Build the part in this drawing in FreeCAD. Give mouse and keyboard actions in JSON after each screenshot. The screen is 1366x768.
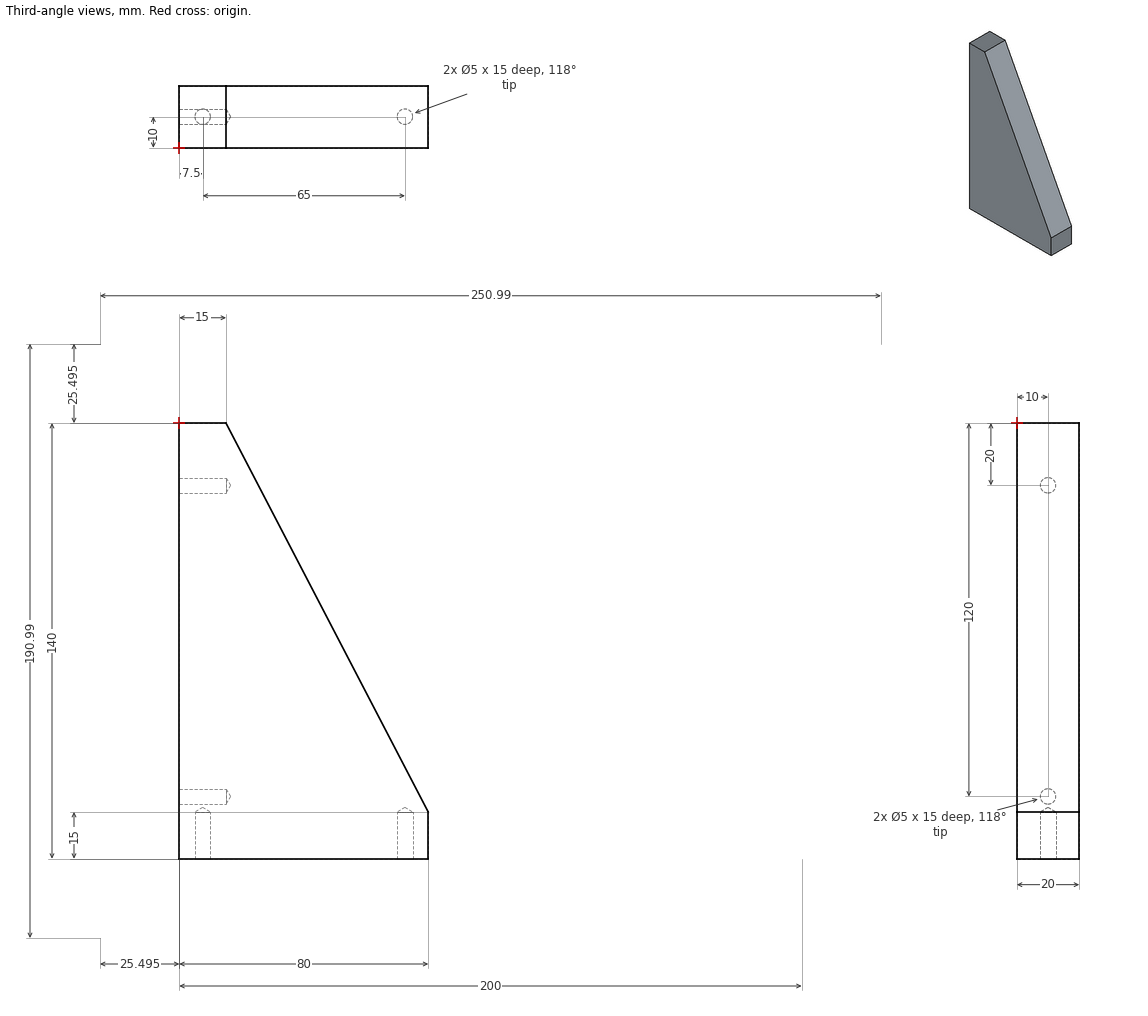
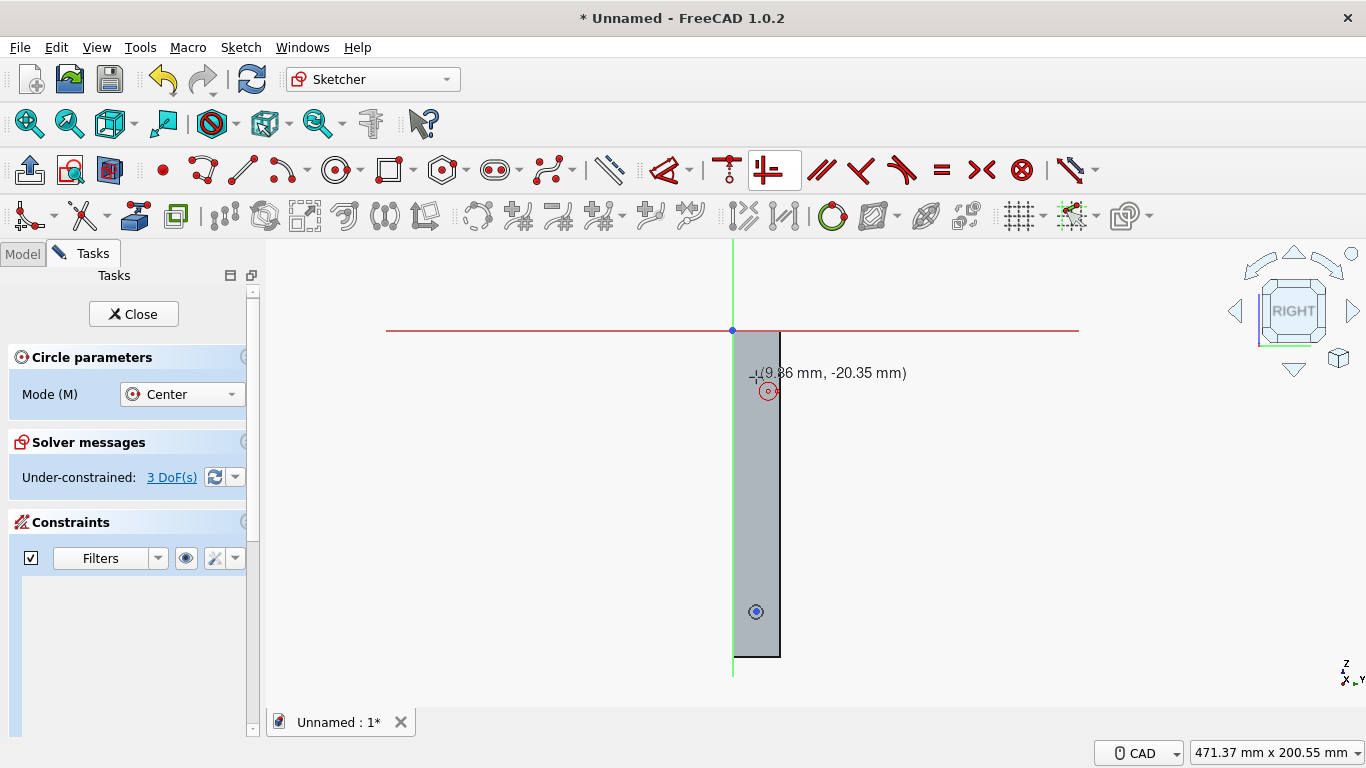
{"action": "left_click", "coordinate": [756, 377]}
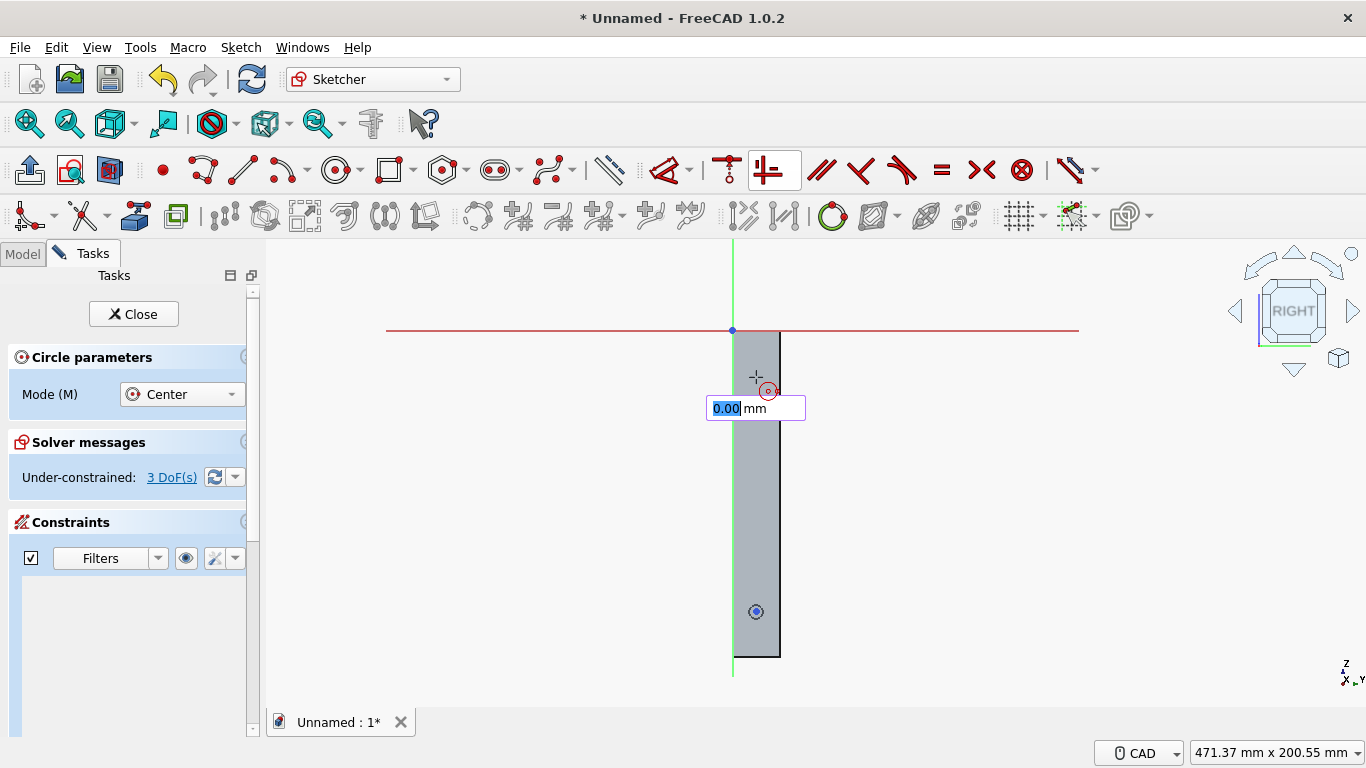
{"action": "scroll", "coordinate": [760, 373], "scroll_direction": "up", "scroll_amount": 6}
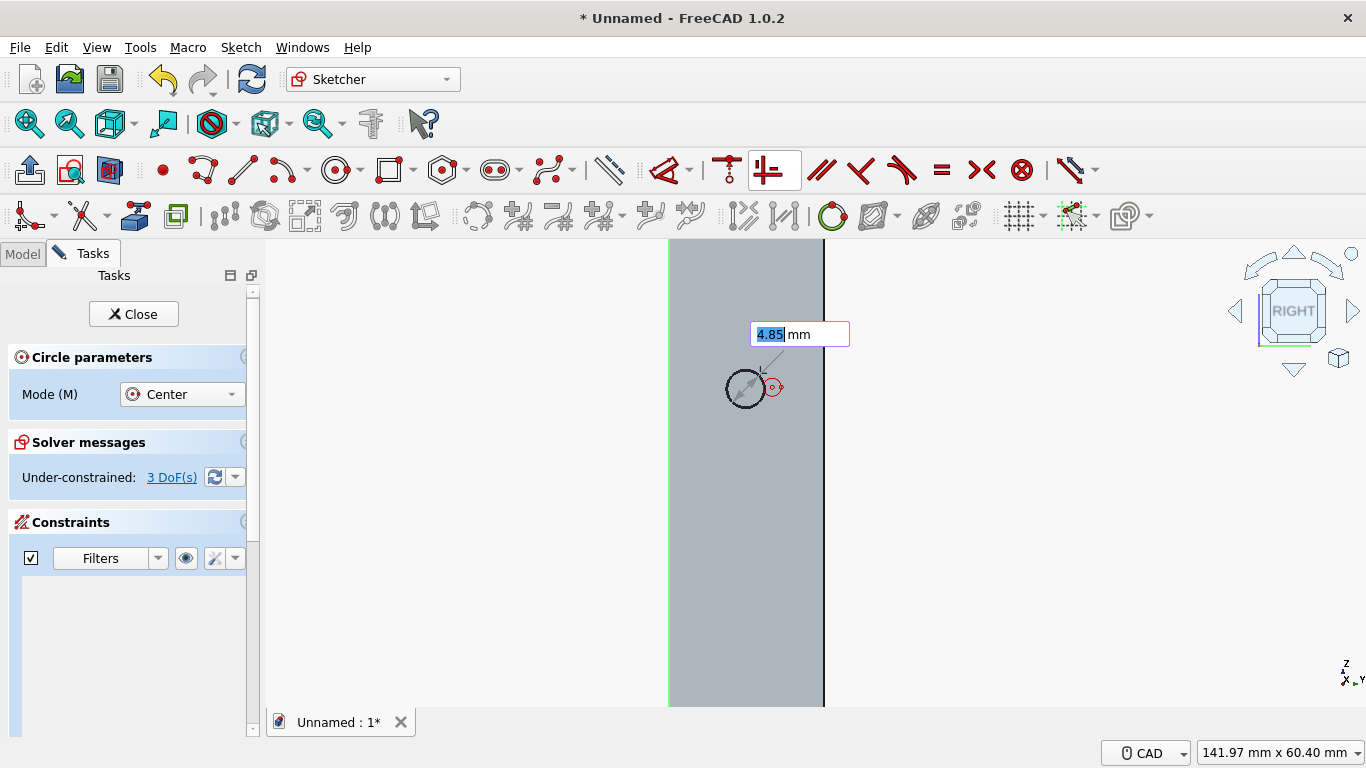
{"action": "left_click", "coordinate": [760, 373]}
{"action": "key", "text": "Escape"}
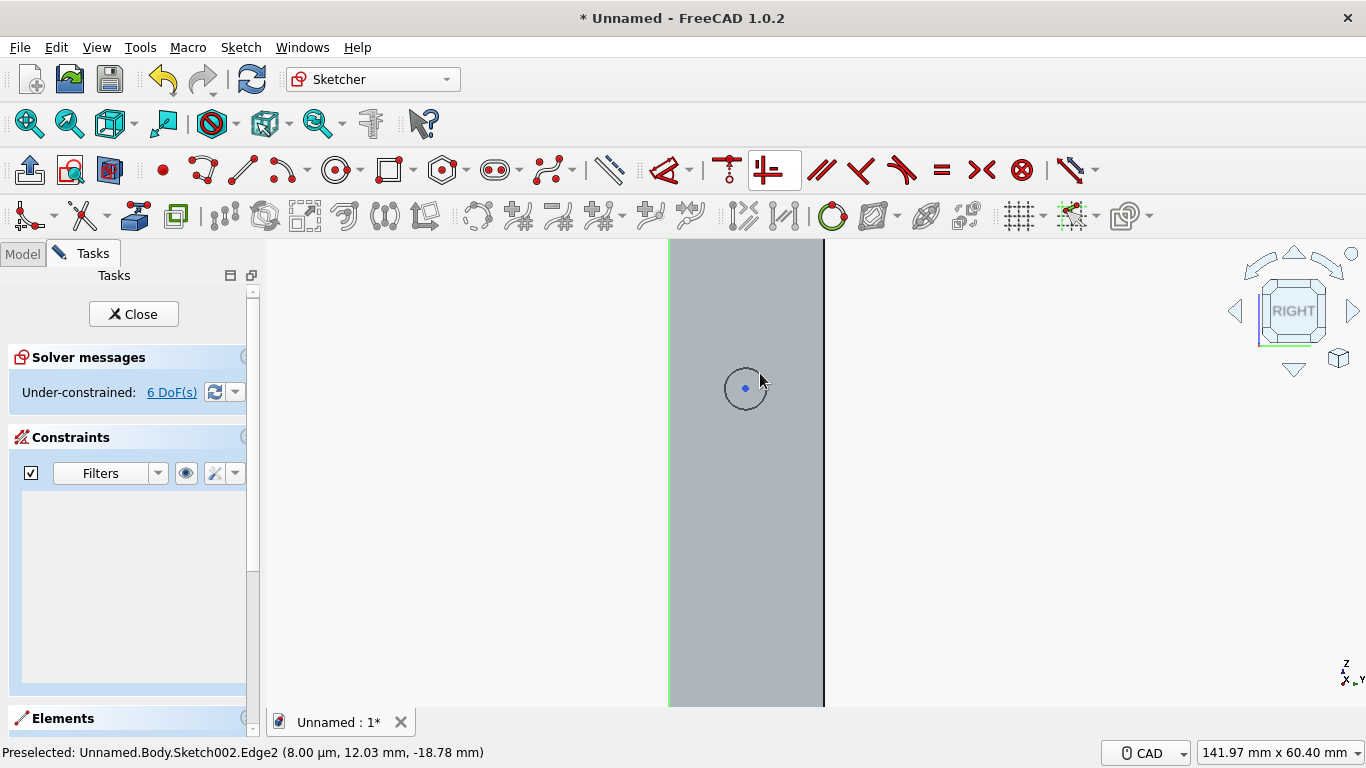
{"action": "scroll", "coordinate": [760, 373], "scroll_direction": "down", "scroll_amount": 6}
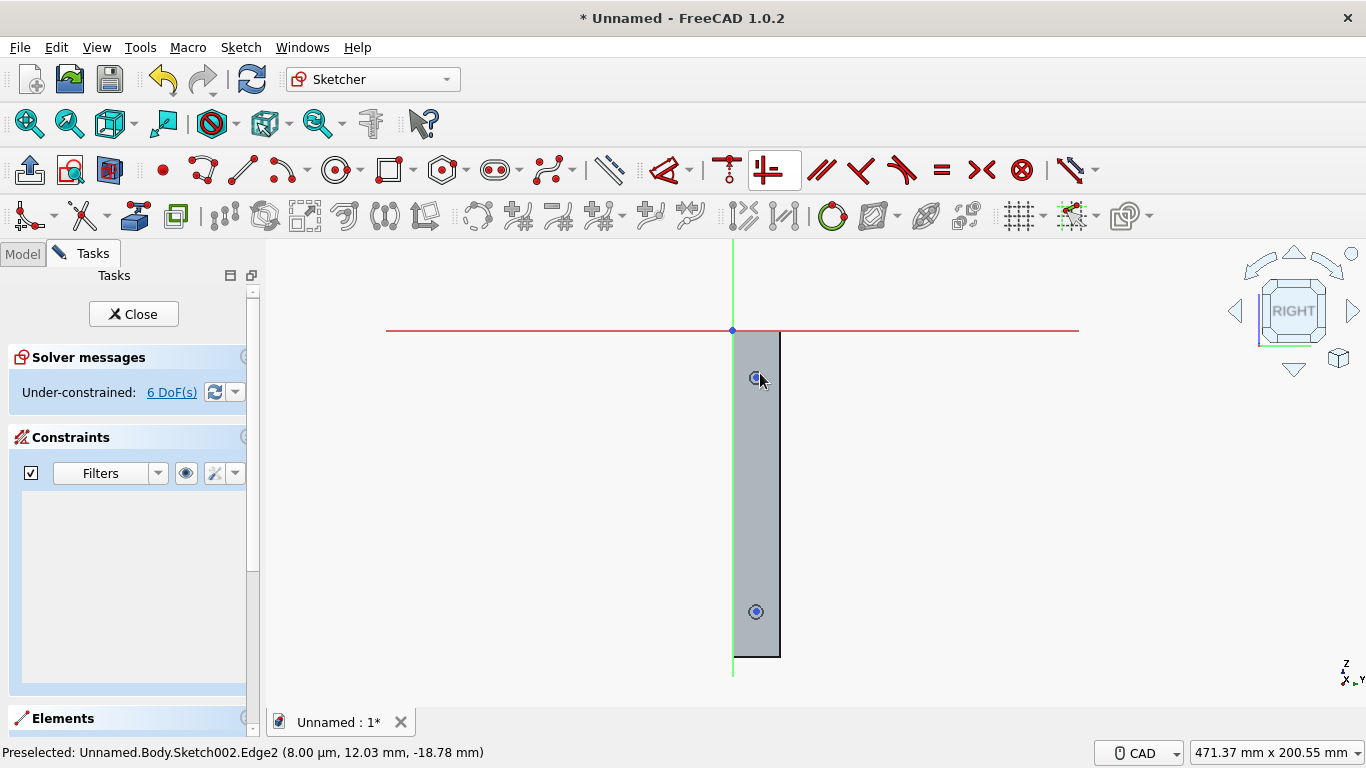
{"action": "scroll", "coordinate": [761, 607], "scroll_direction": "up", "scroll_amount": 4}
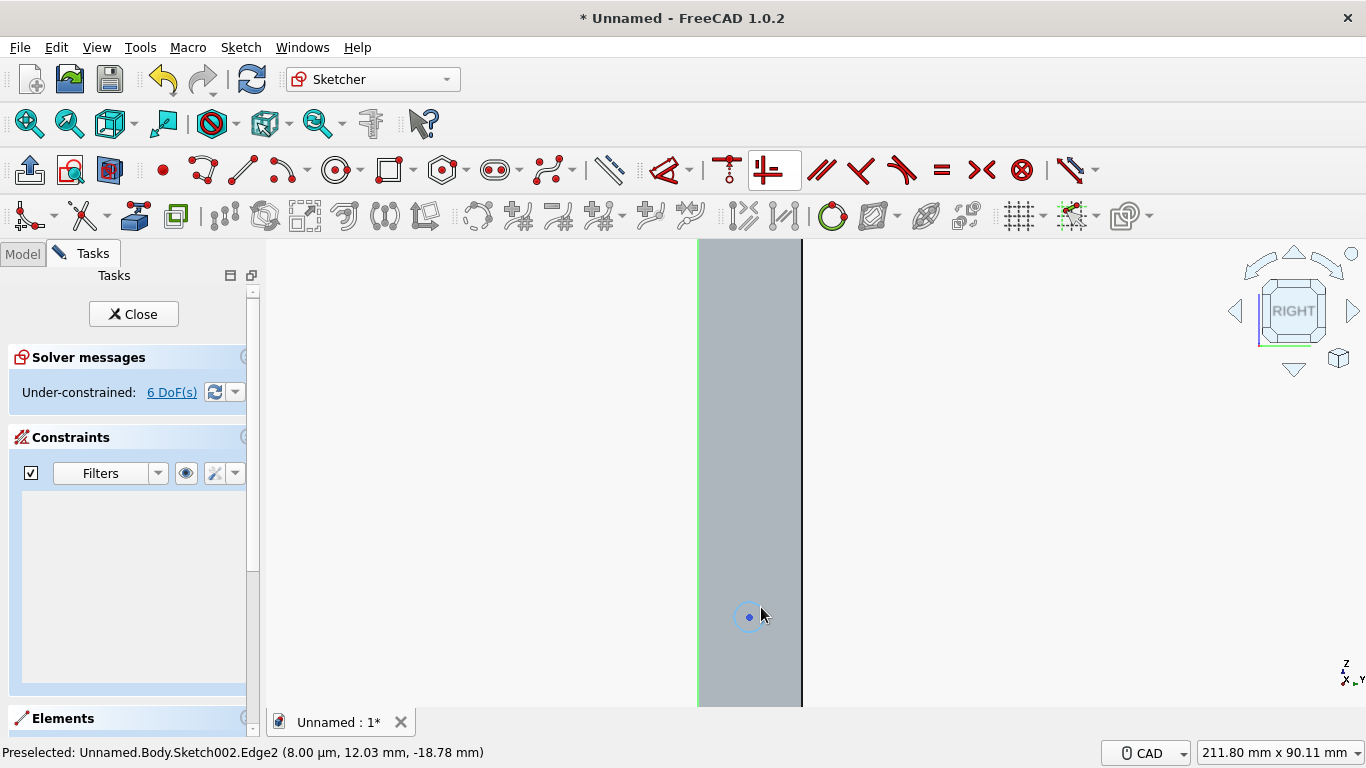
{"action": "left_click", "coordinate": [760, 607]}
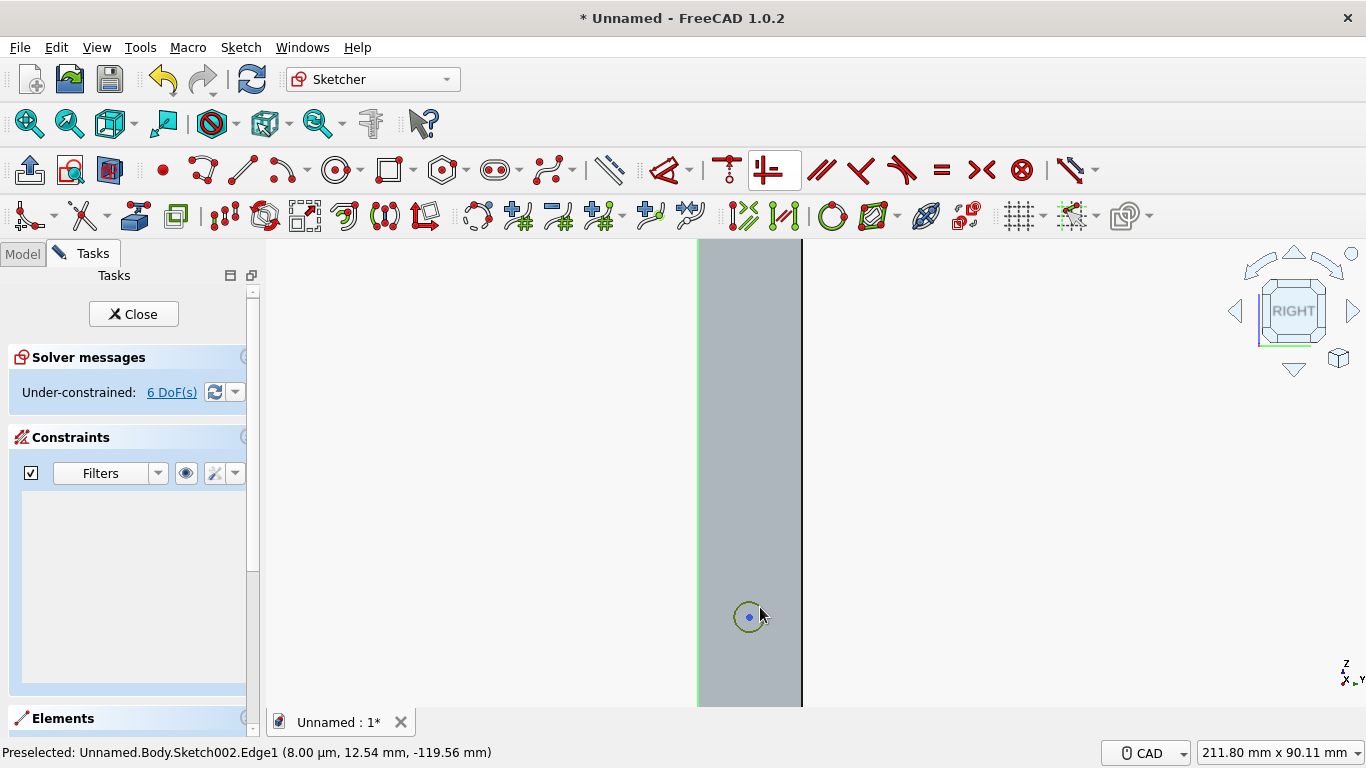
{"action": "scroll", "coordinate": [761, 607], "scroll_direction": "down", "scroll_amount": 4}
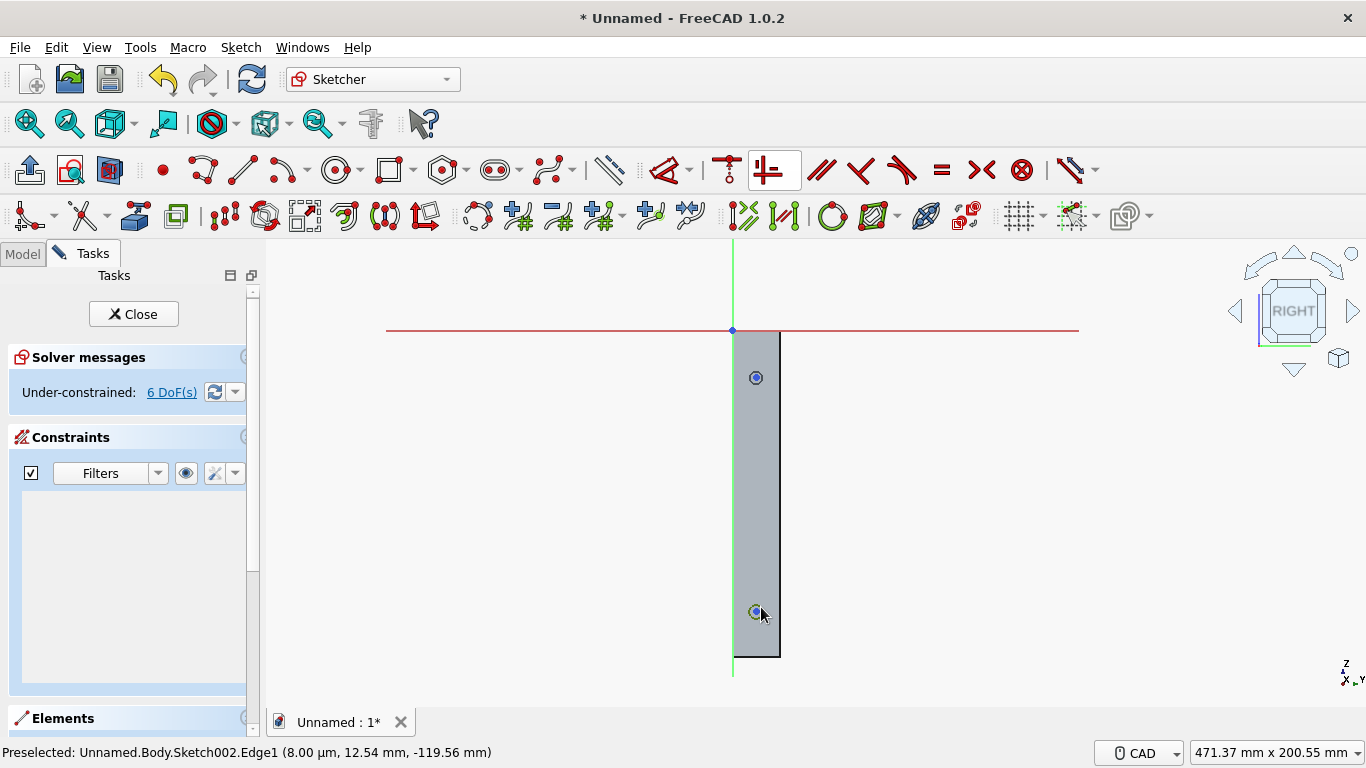
{"action": "scroll", "coordinate": [760, 374], "scroll_direction": "up", "scroll_amount": 4}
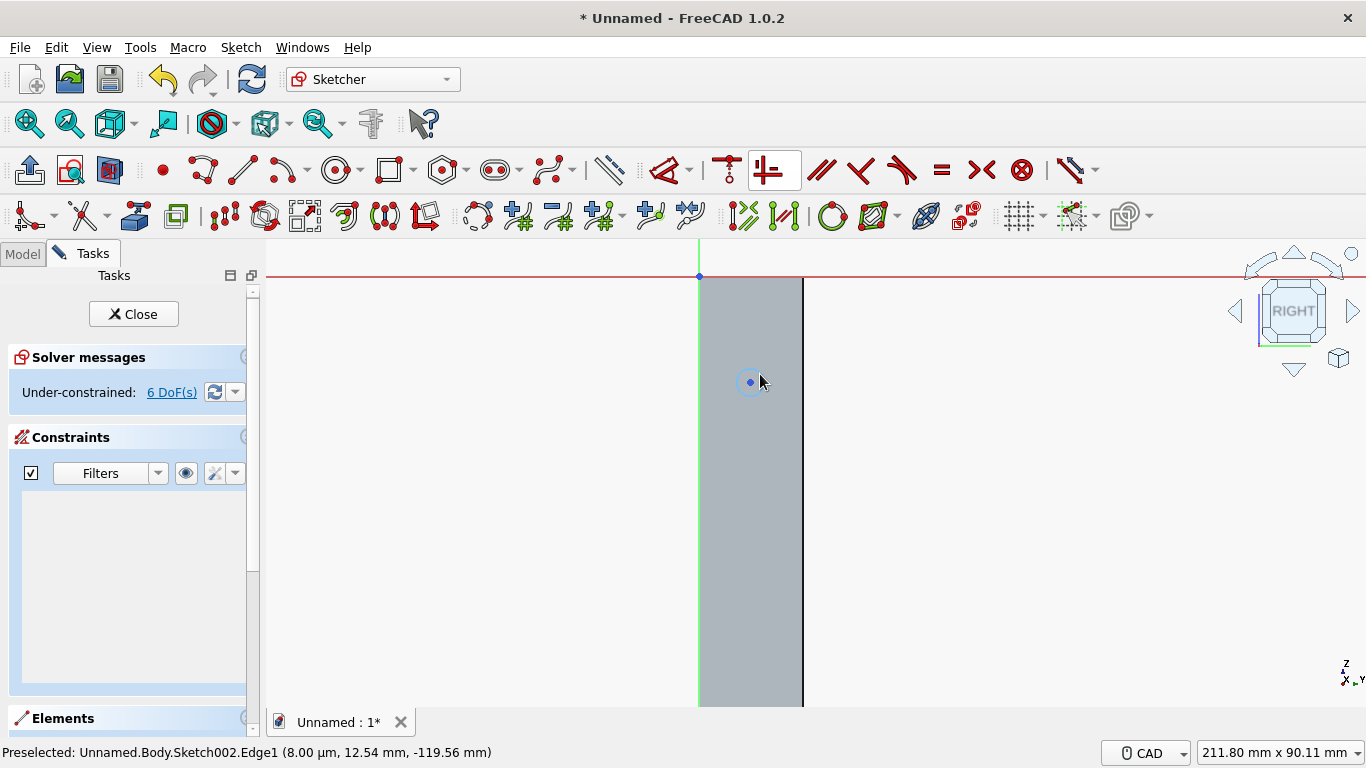
{"action": "left_click", "coordinate": [760, 373]}